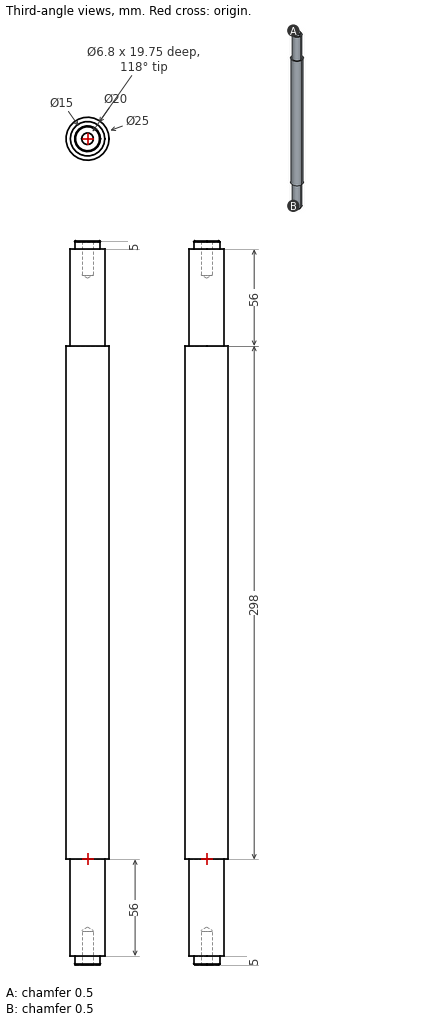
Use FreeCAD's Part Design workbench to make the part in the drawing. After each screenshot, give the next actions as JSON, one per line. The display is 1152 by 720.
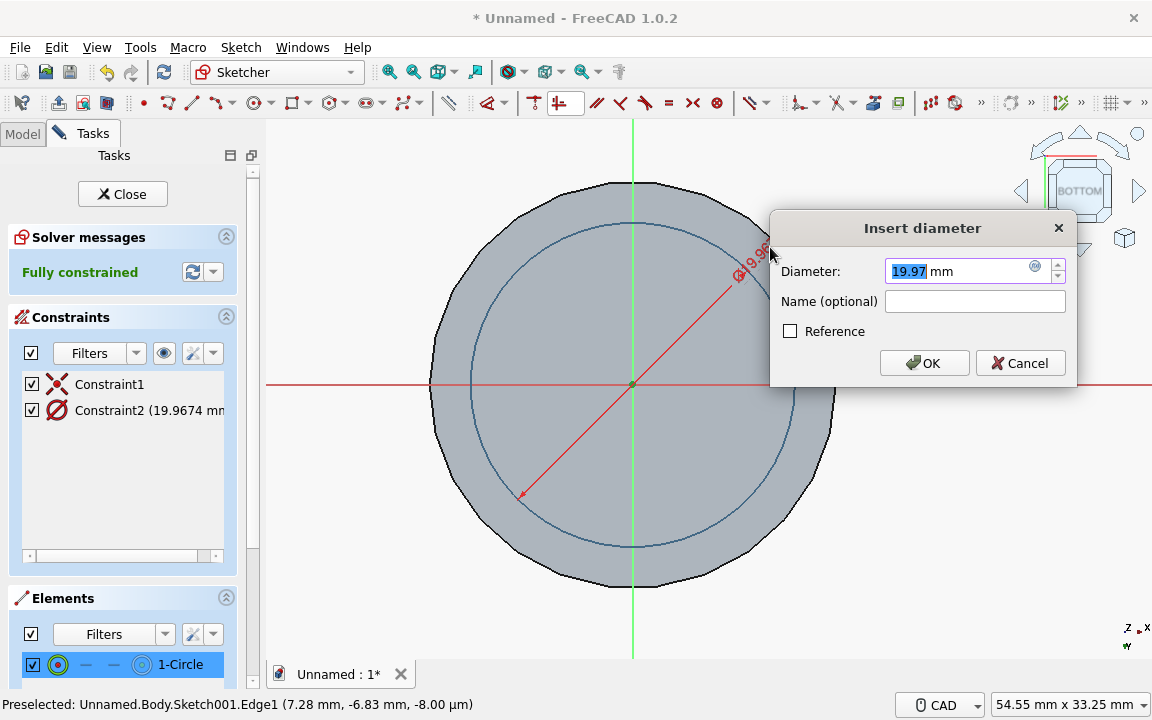
{"action": "type", "text": "20"}
{"action": "key", "text": "Return"}
{"action": "key", "text": "Escape"}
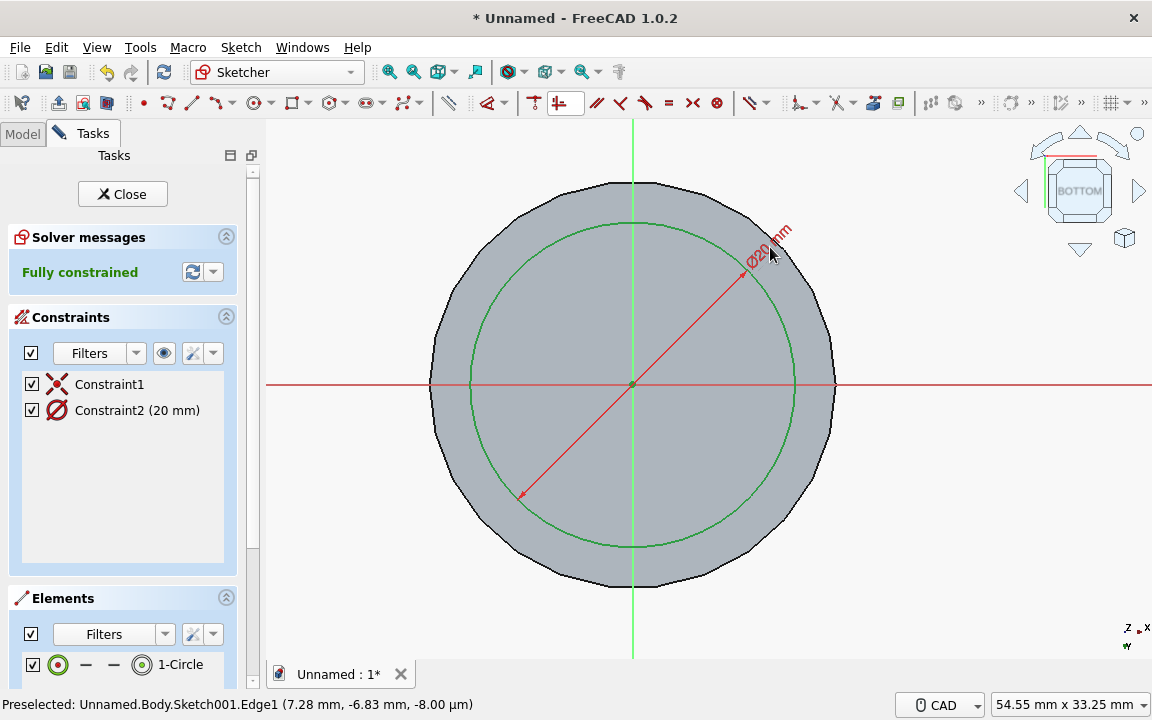
{"action": "left_click", "coordinate": [123, 194]}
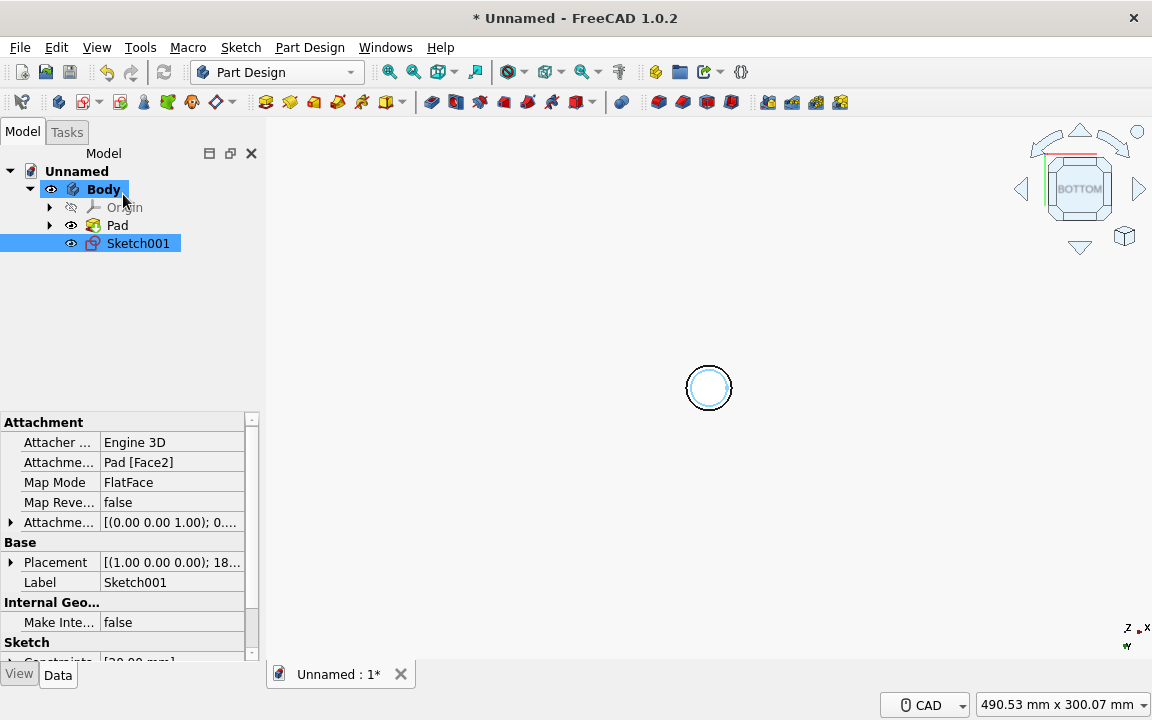
{"action": "left_click", "coordinate": [266, 102]}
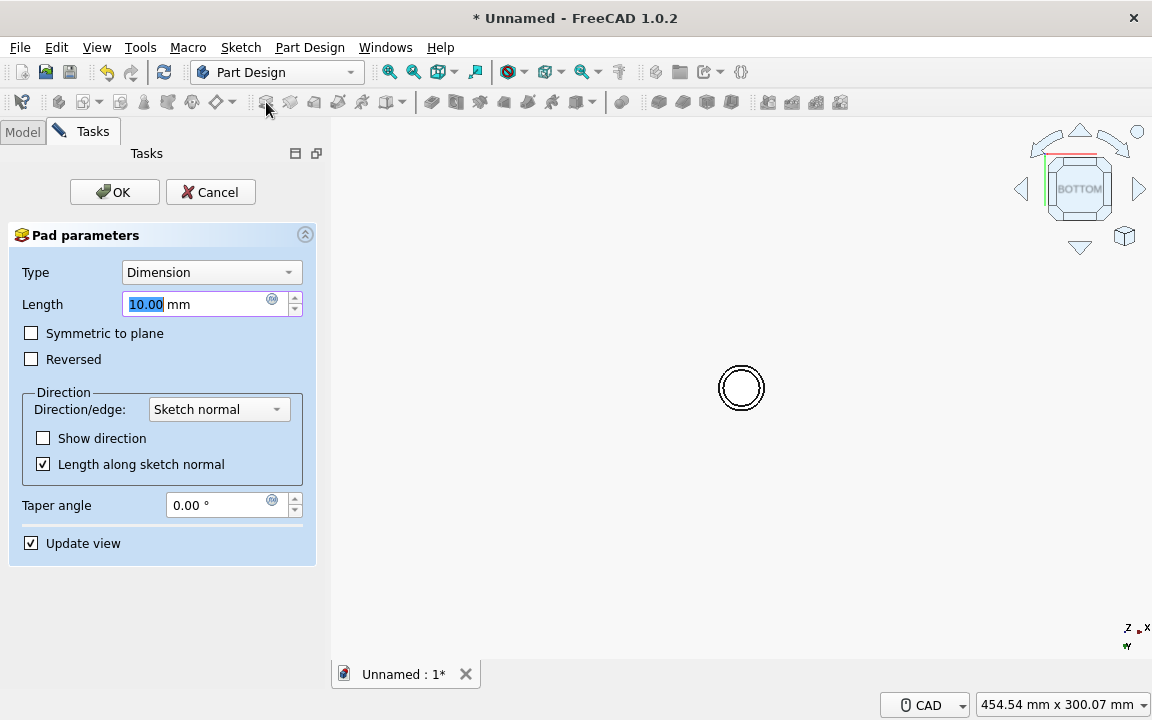
{"action": "type", "text": "56"}
{"action": "key", "text": "Tab"}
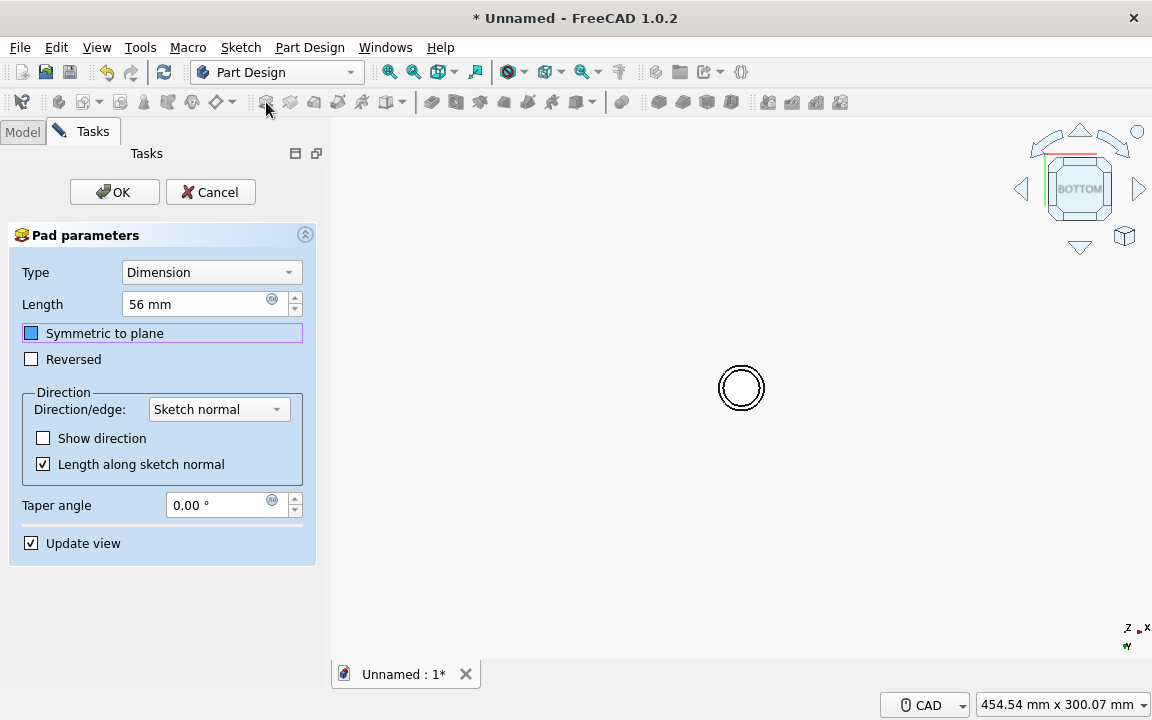
{"action": "left_click", "coordinate": [115, 192]}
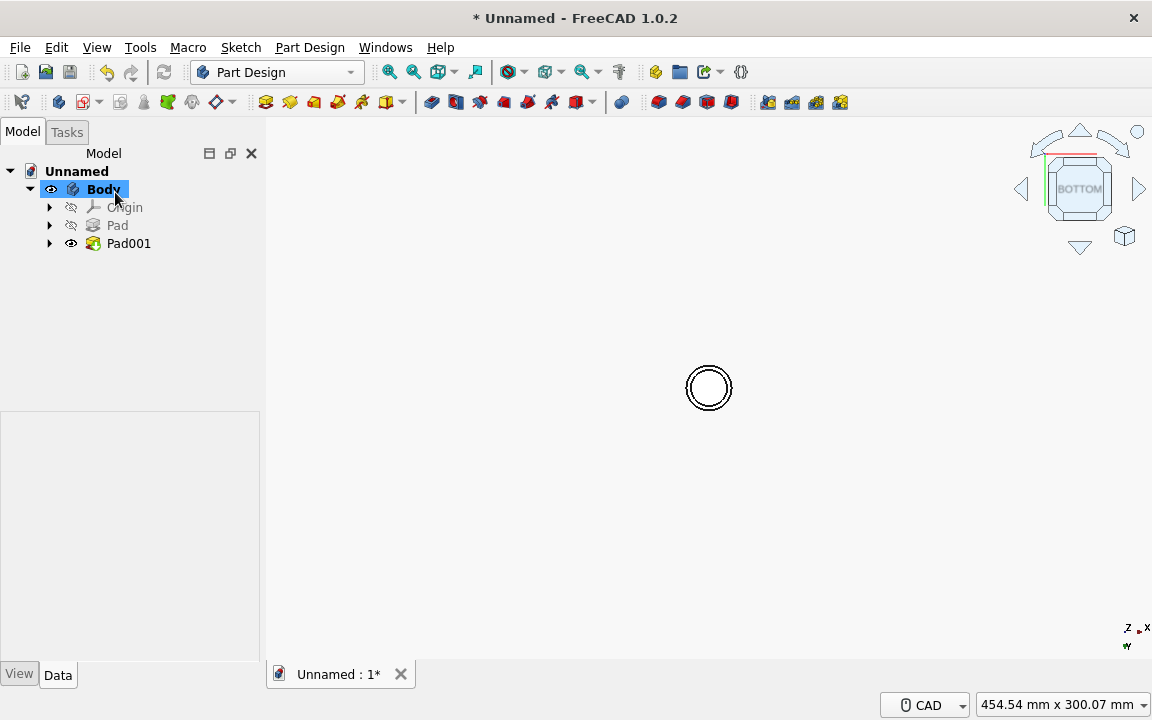
{"action": "left_click", "coordinate": [390, 72]}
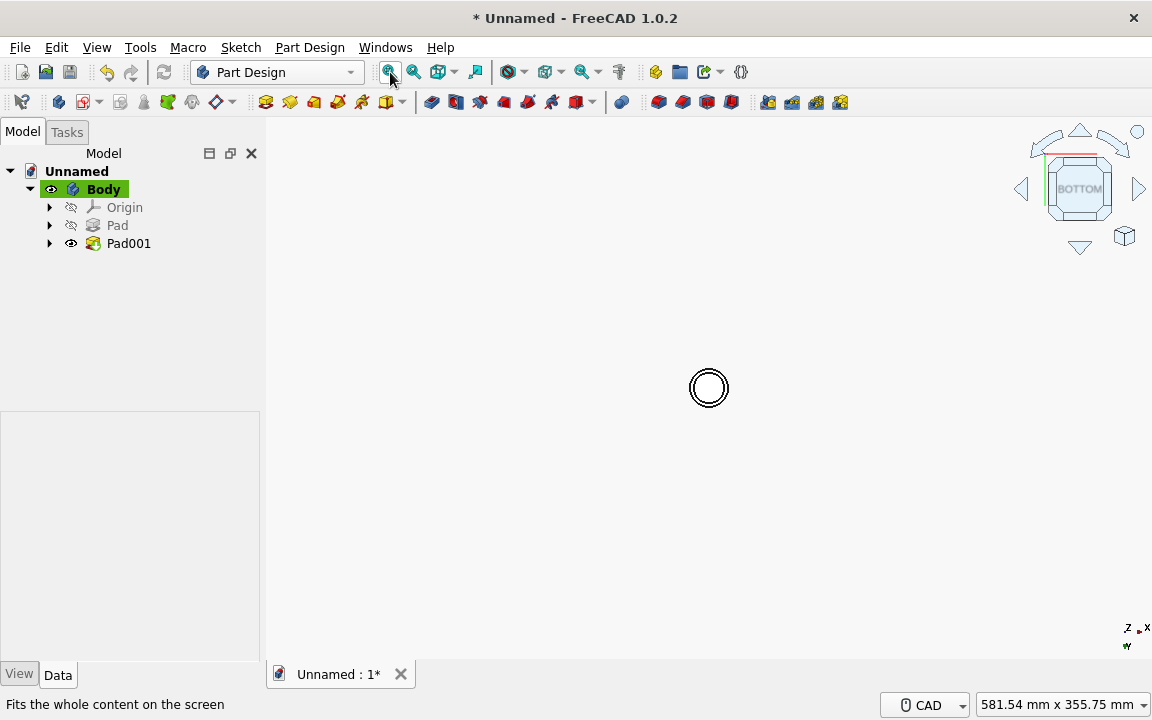
{"action": "left_click", "coordinate": [50, 207]}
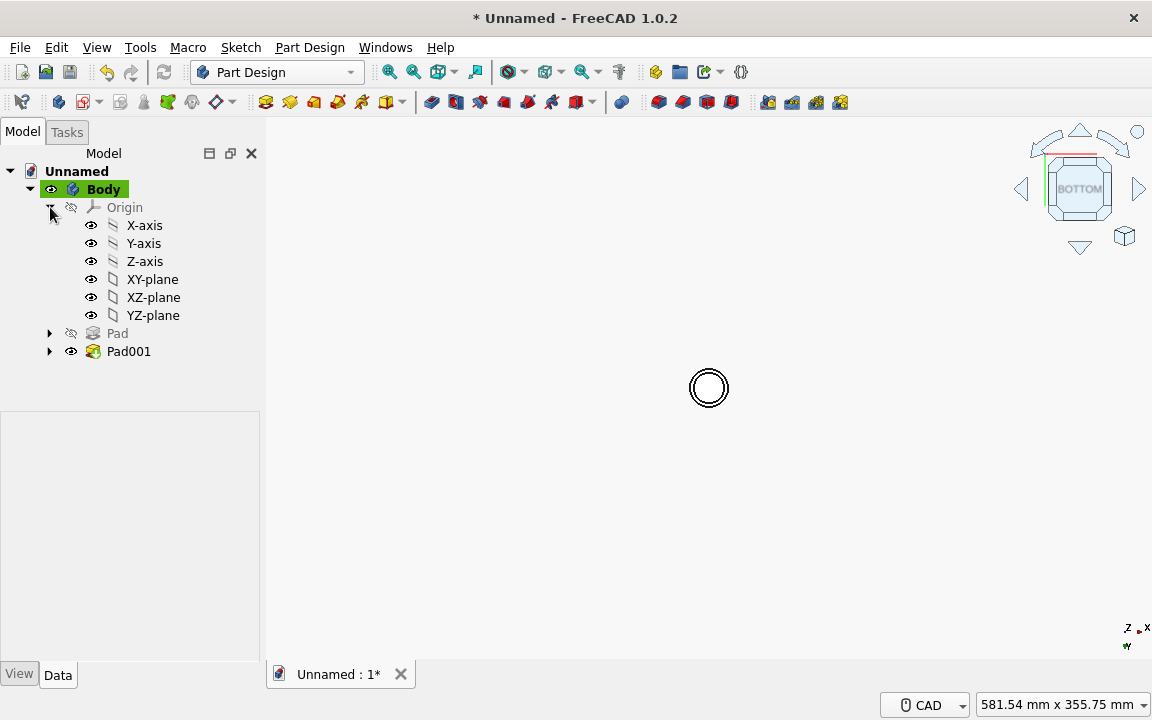
{"action": "left_click", "coordinate": [136, 279]}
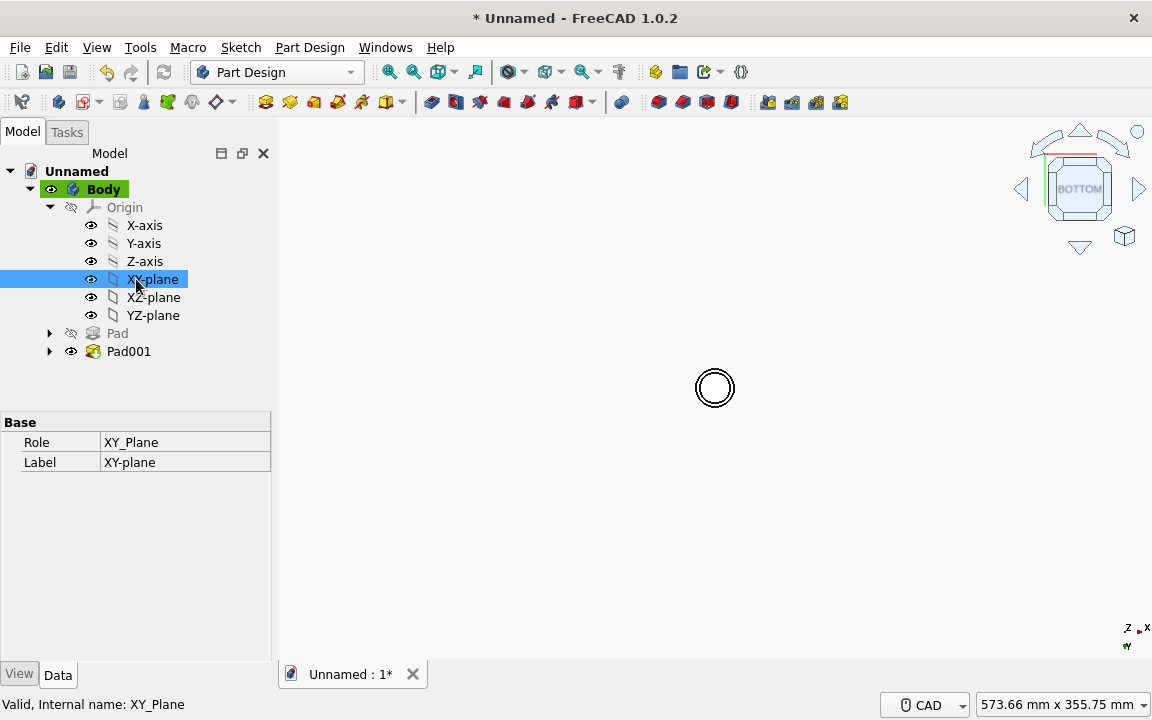
{"action": "left_click", "coordinate": [216, 102]}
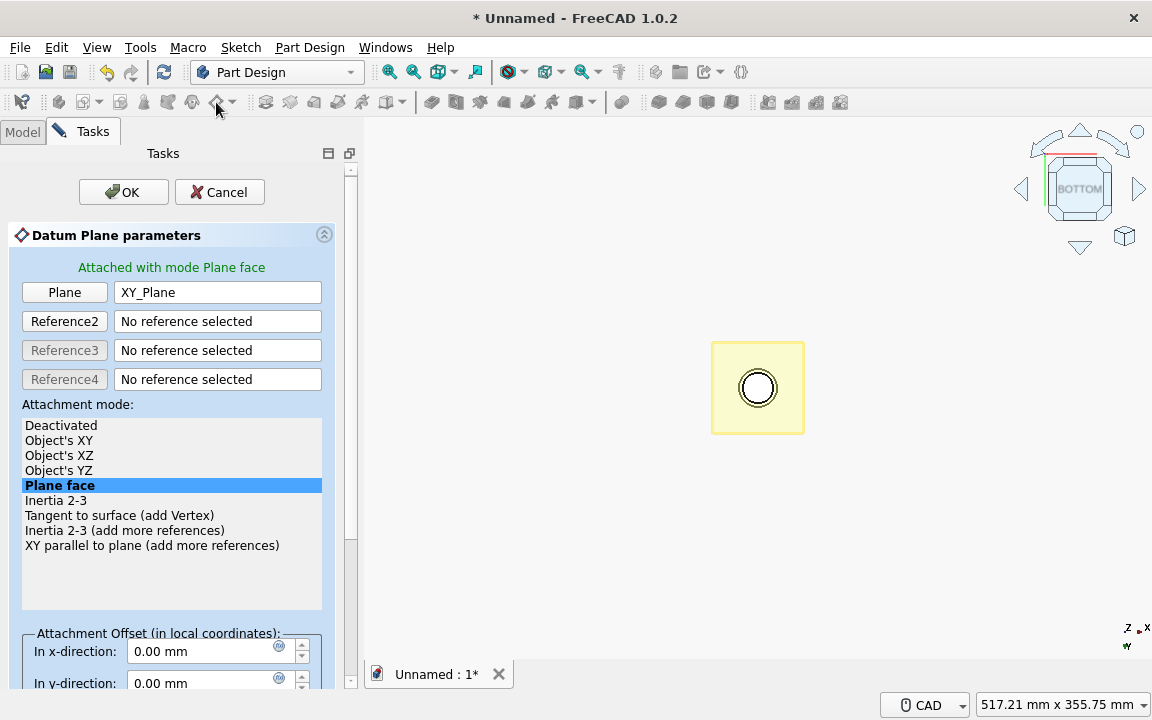
{"action": "scroll", "coordinate": [351, 426], "scroll_direction": "down", "scroll_amount": 2}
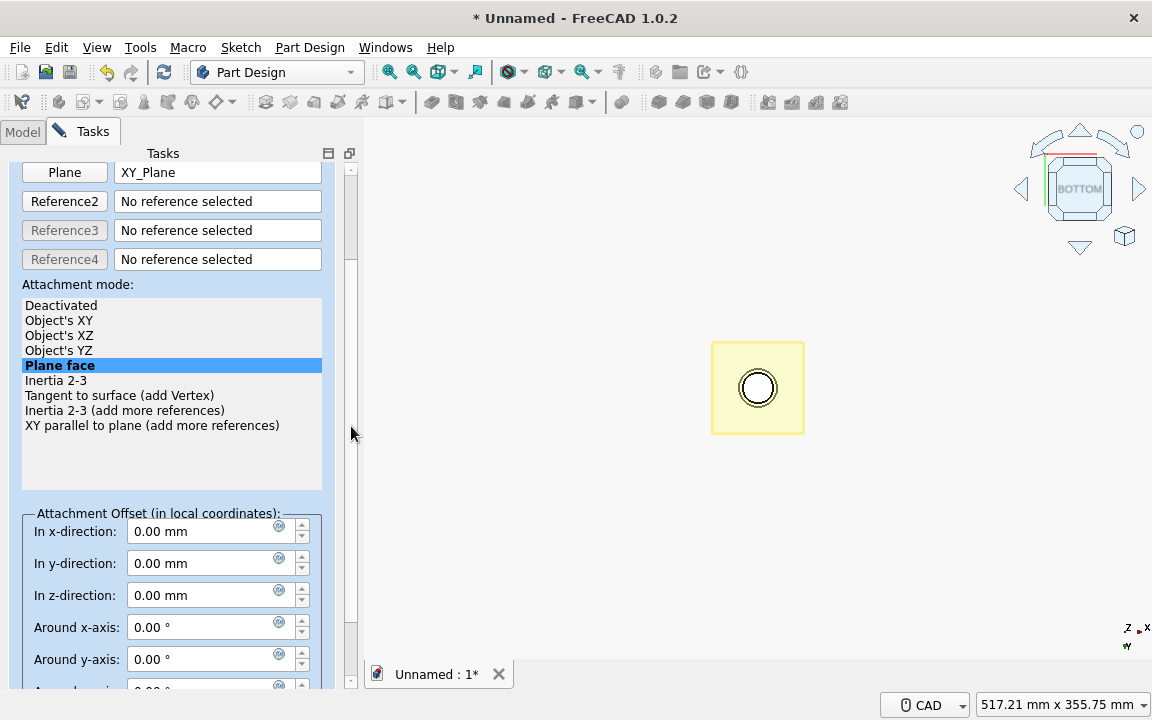
{"action": "triple_click", "coordinate": [210, 595]}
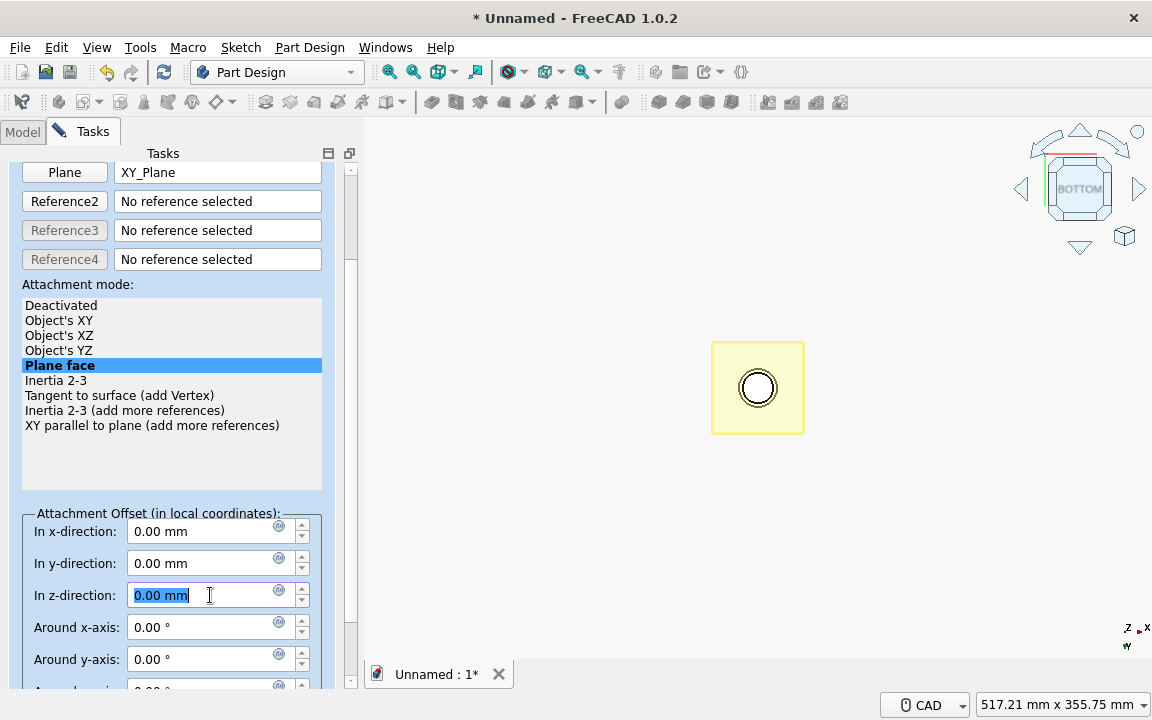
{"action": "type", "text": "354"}
{"action": "key", "text": "Tab"}